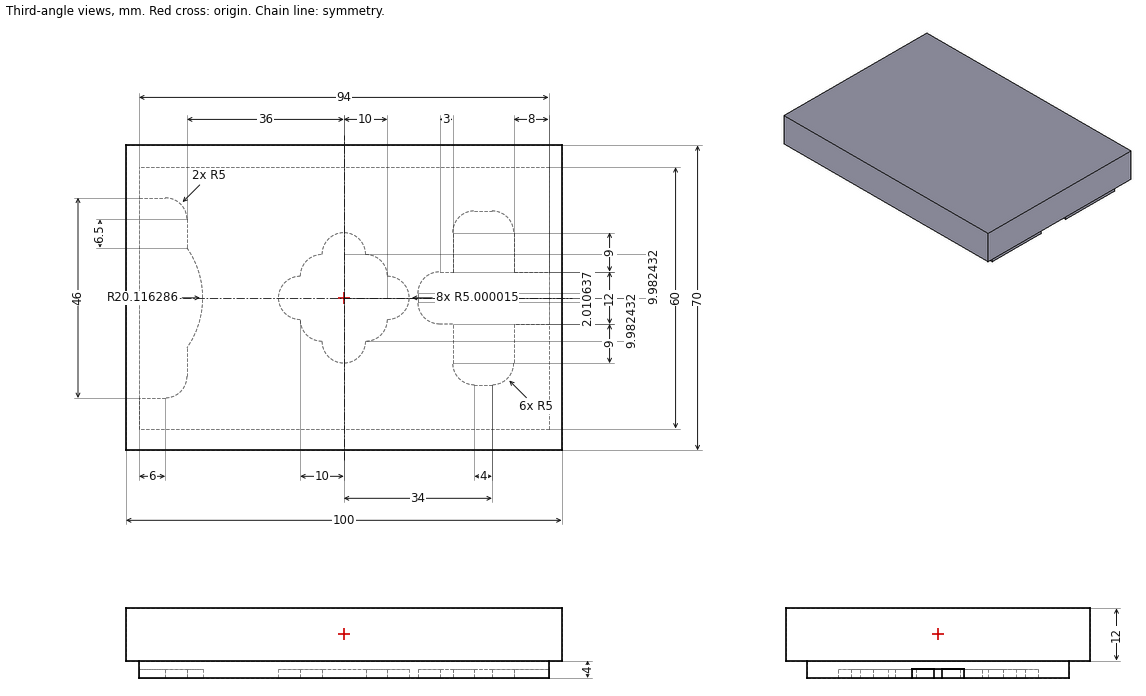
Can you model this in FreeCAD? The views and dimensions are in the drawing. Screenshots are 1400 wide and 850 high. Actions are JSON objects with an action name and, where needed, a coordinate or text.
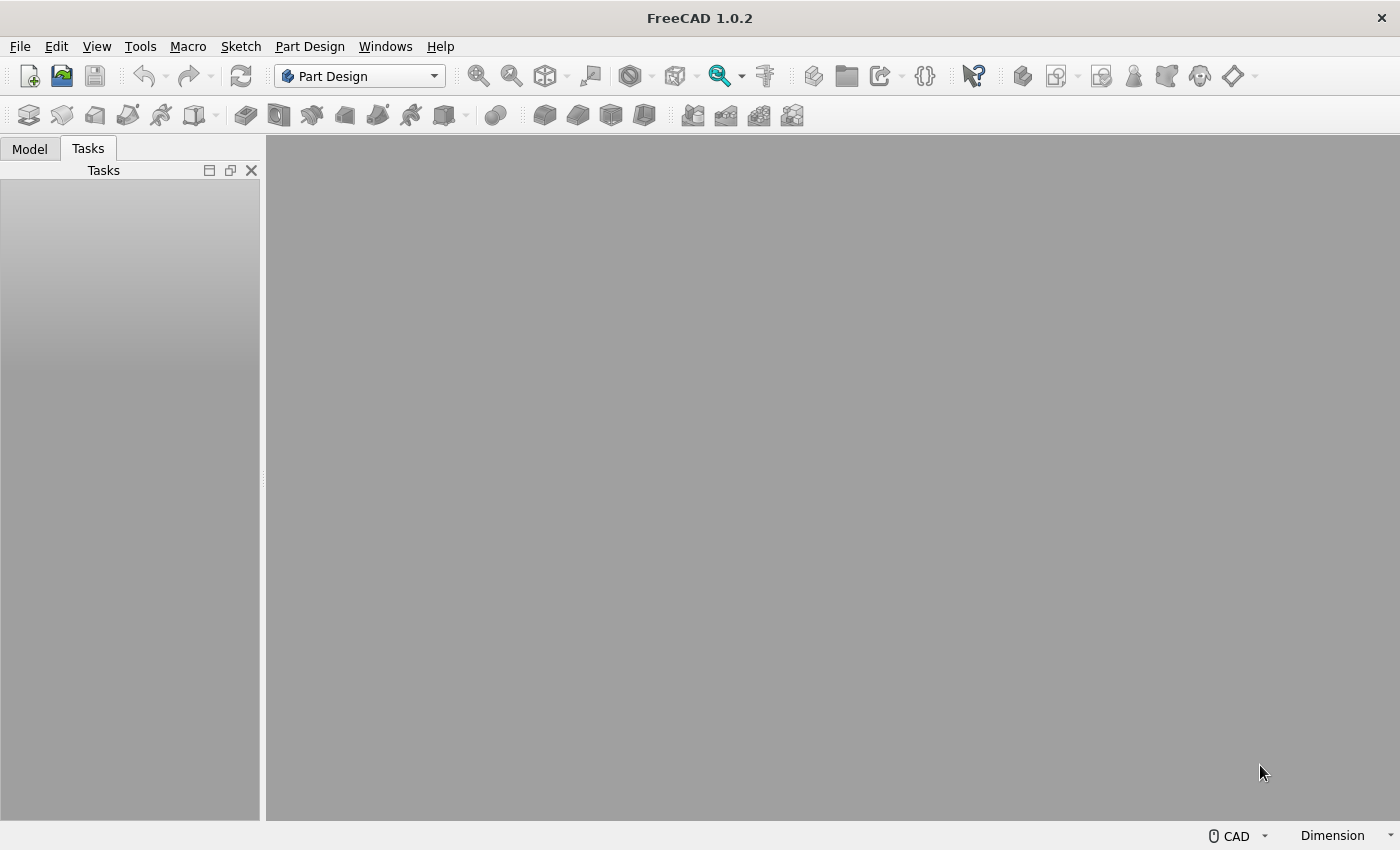
{"action": "left_click", "coordinate": [29, 76]}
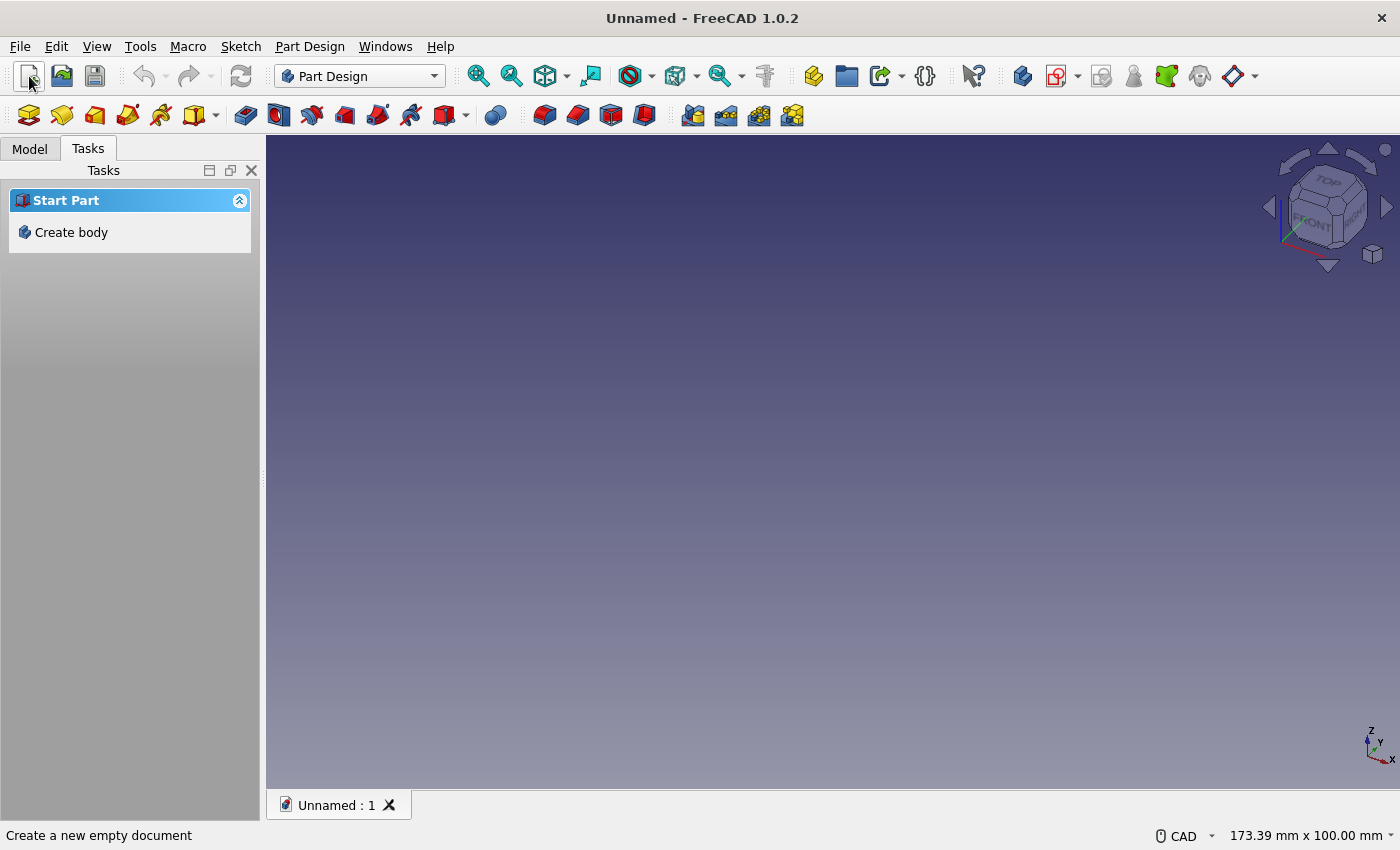
{"action": "left_click", "coordinate": [1056, 76]}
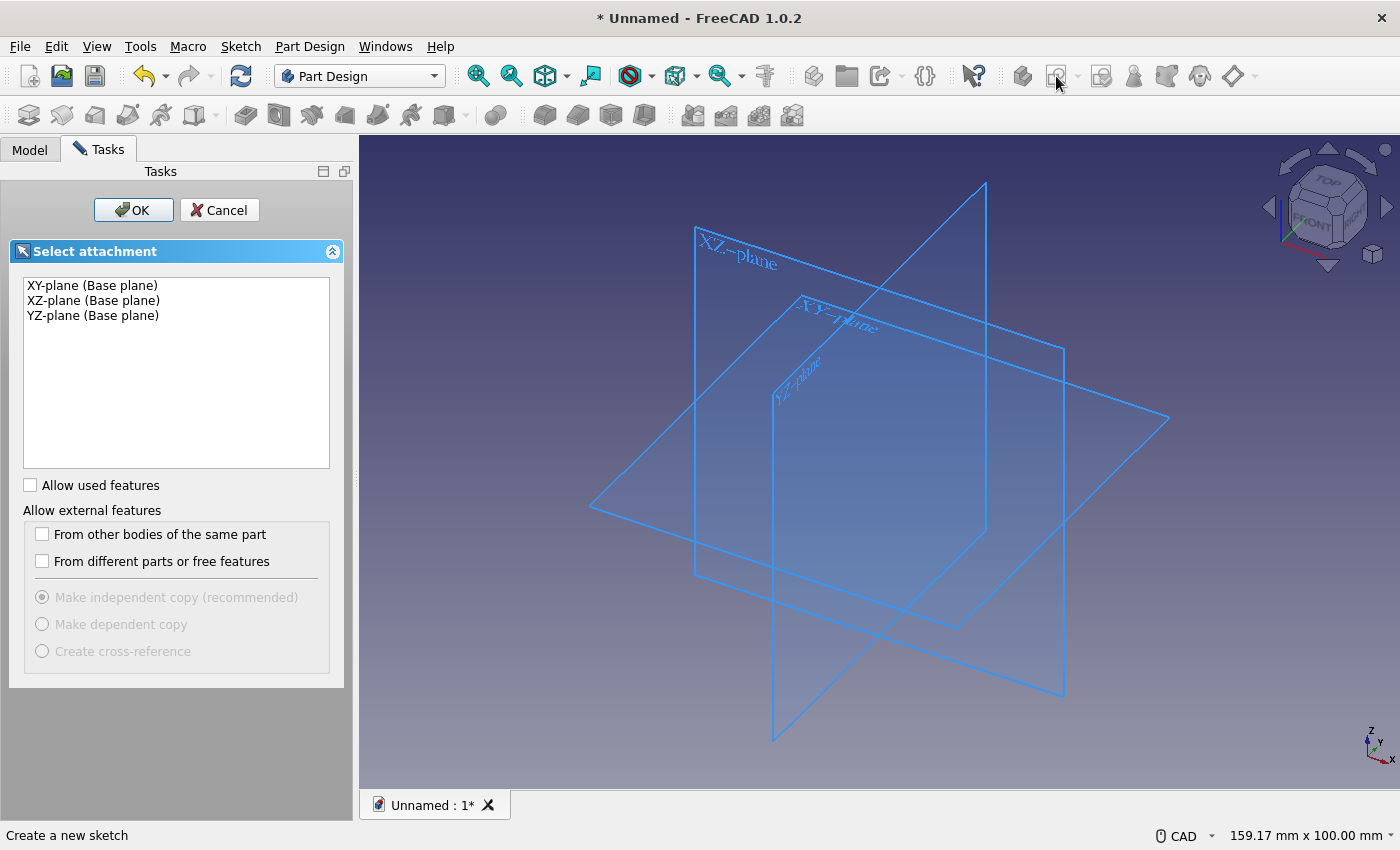
{"action": "left_click", "coordinate": [84, 286]}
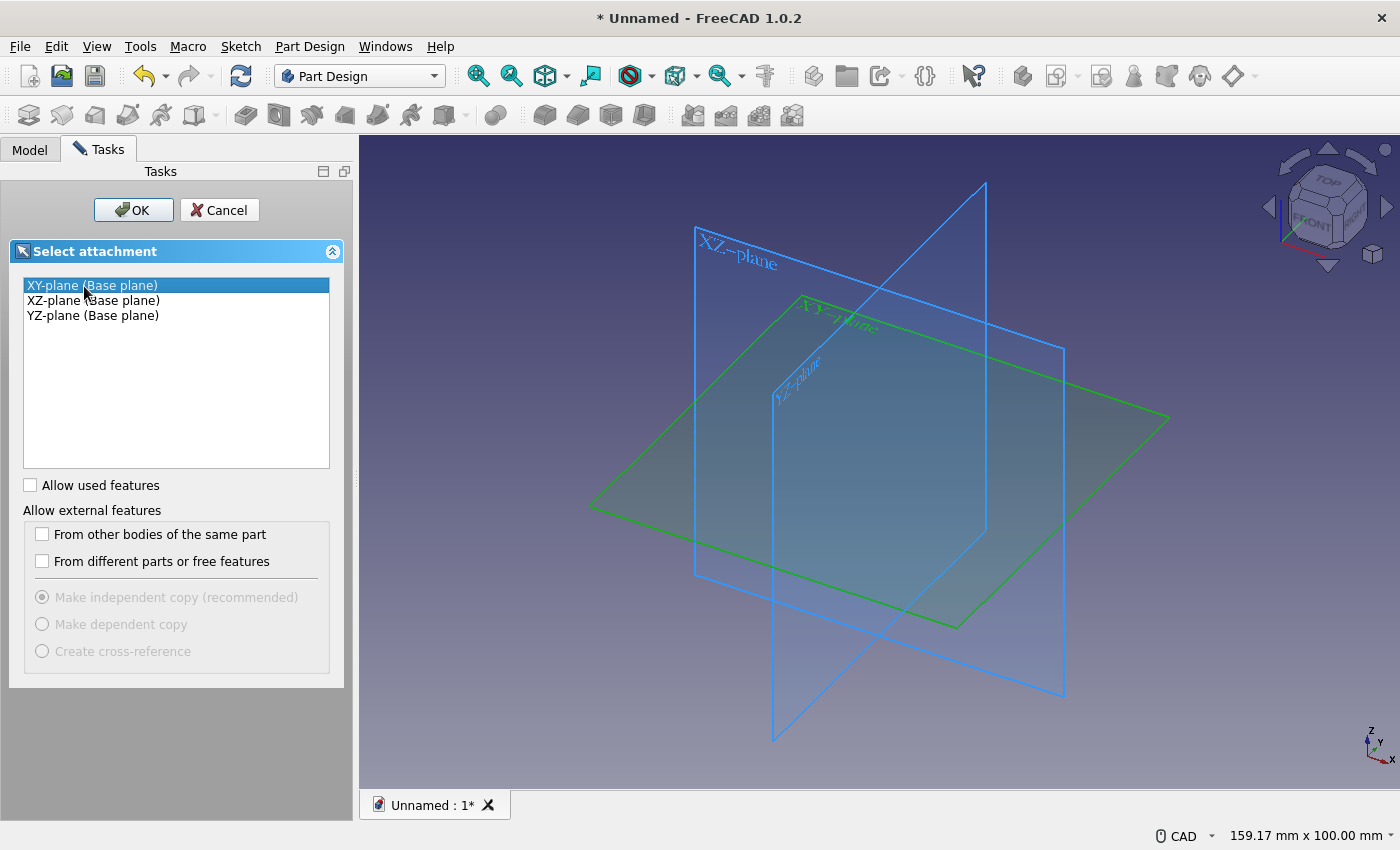
{"action": "left_click", "coordinate": [134, 210]}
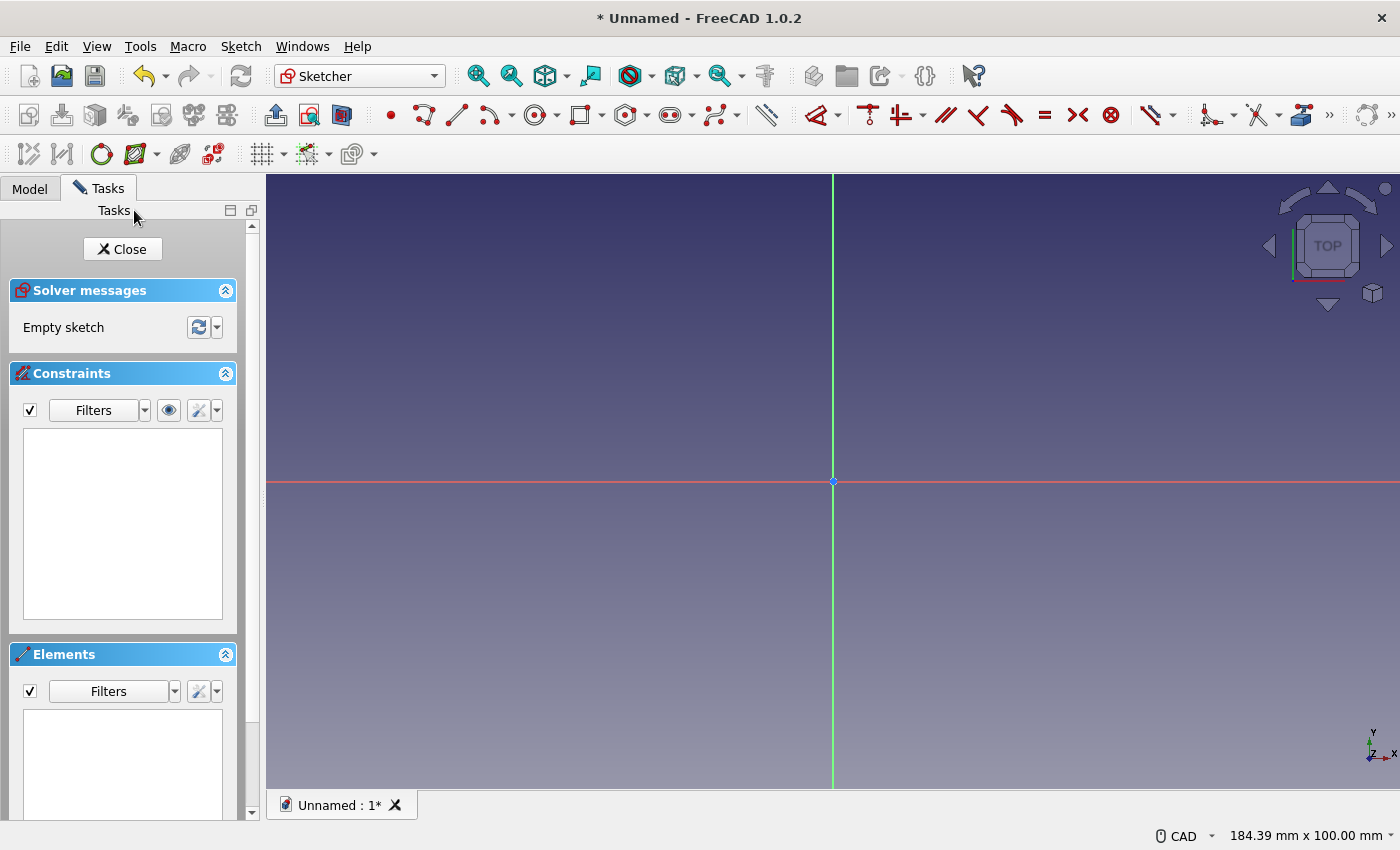
{"action": "left_click", "coordinate": [602, 116]}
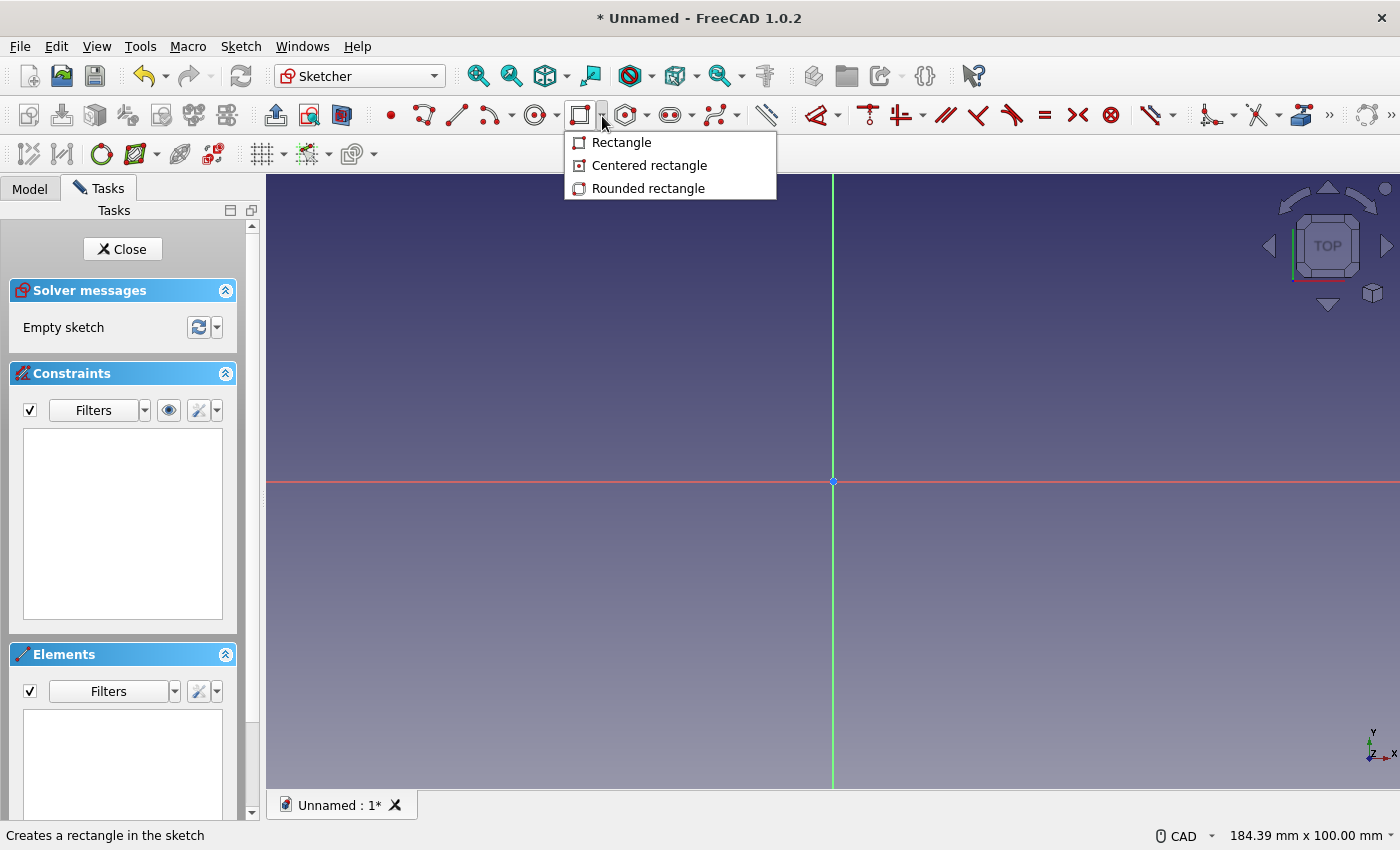
{"action": "left_click", "coordinate": [670, 166]}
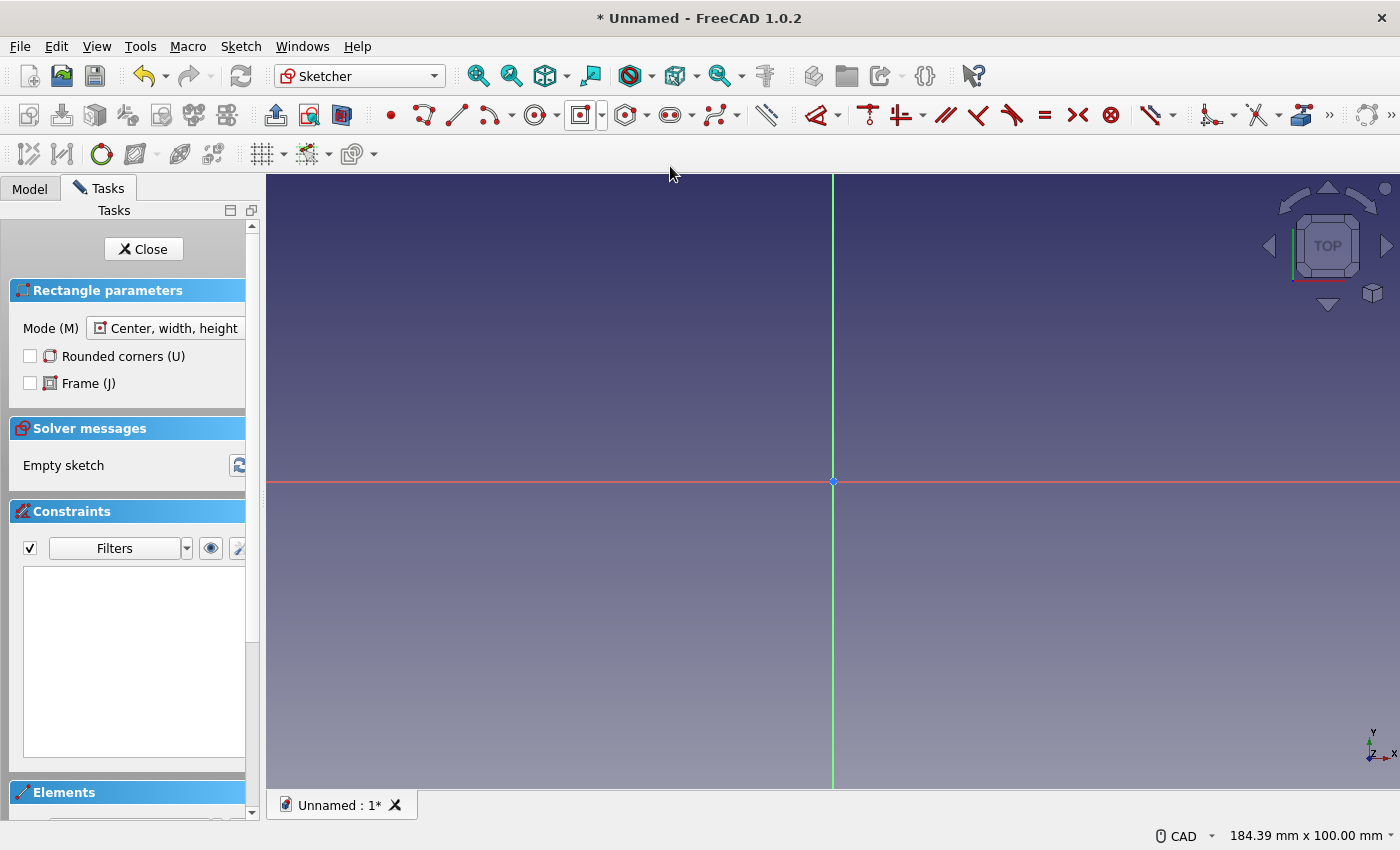
{"action": "left_click", "coordinate": [833, 482]}
{"action": "mouse_move", "coordinate": [1140, 266]}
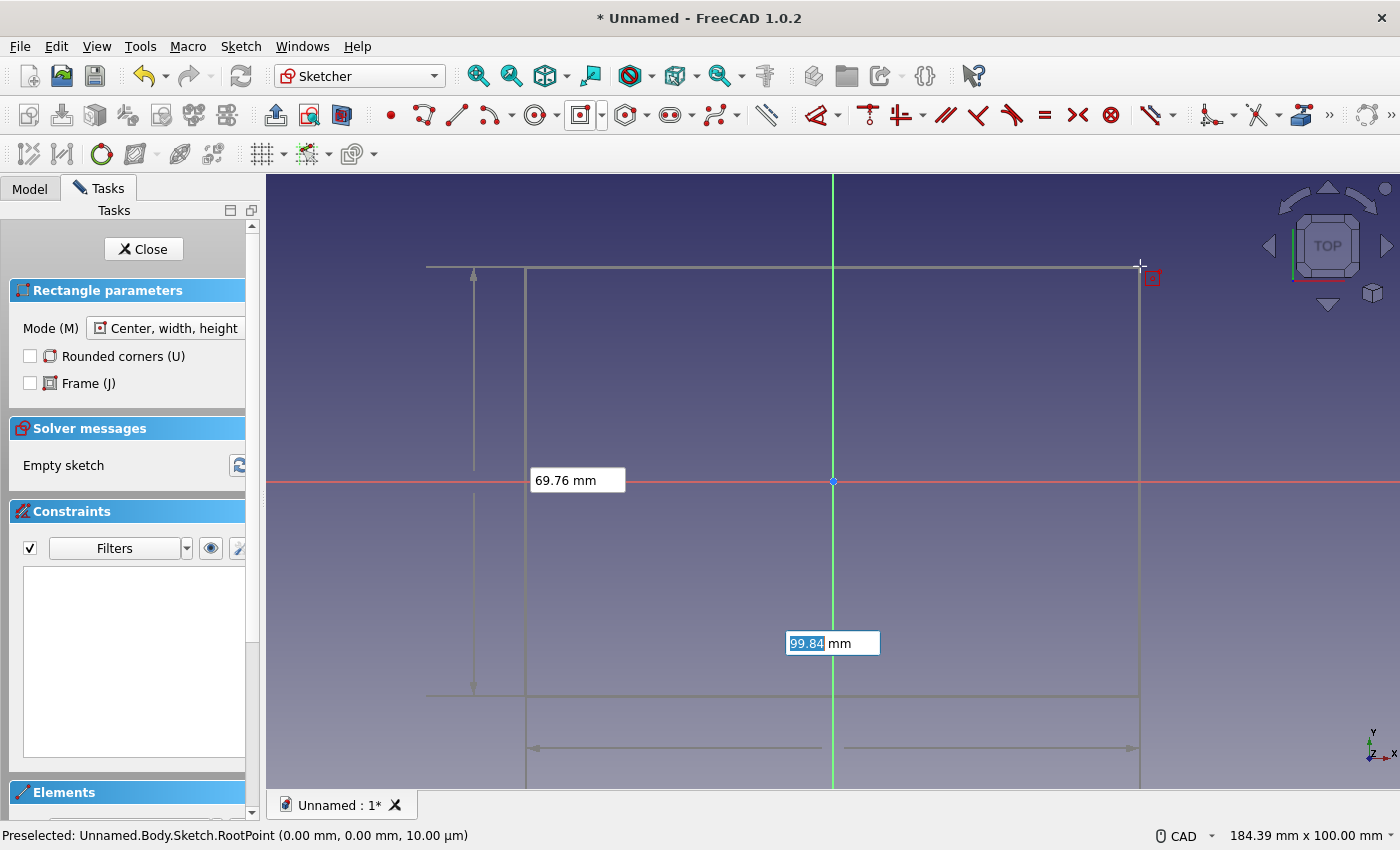
{"action": "type", "text": "100"}
{"action": "key", "text": "Tab"}
{"action": "type", "text": "70"}
{"action": "key", "text": "Return"}
{"action": "key", "text": "Escape"}